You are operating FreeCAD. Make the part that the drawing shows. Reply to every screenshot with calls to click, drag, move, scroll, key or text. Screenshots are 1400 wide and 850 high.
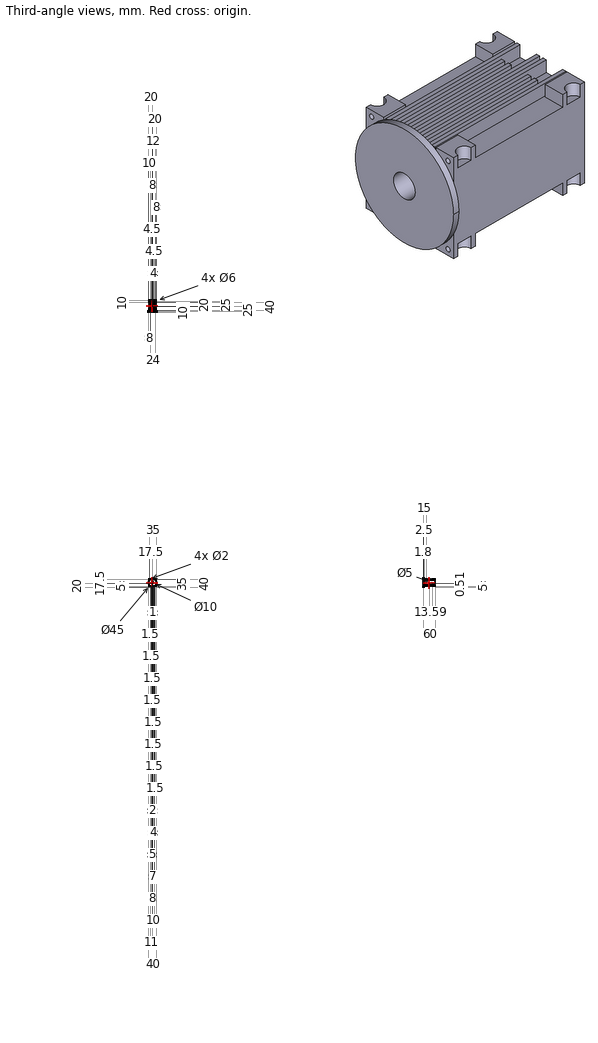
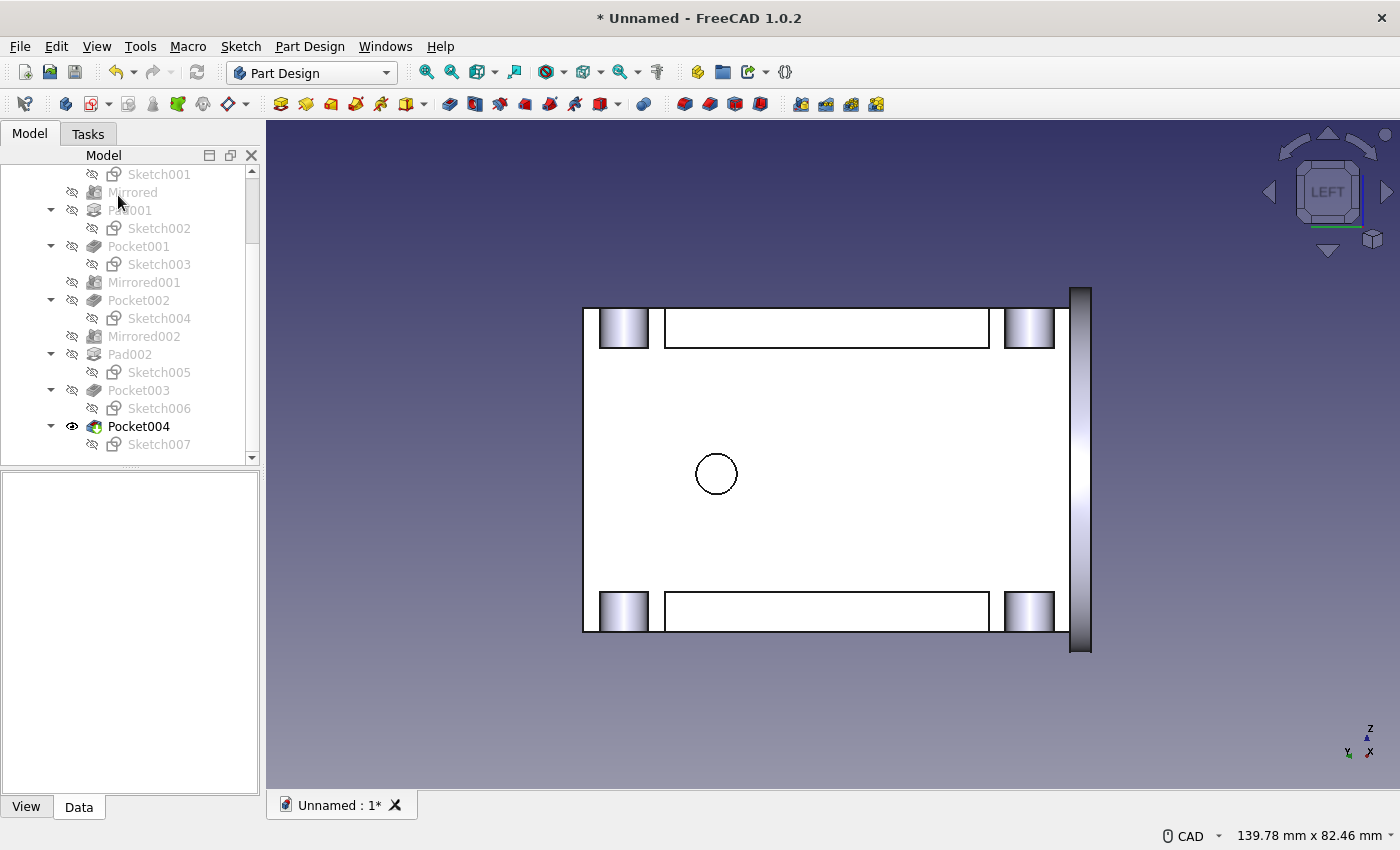
key(4)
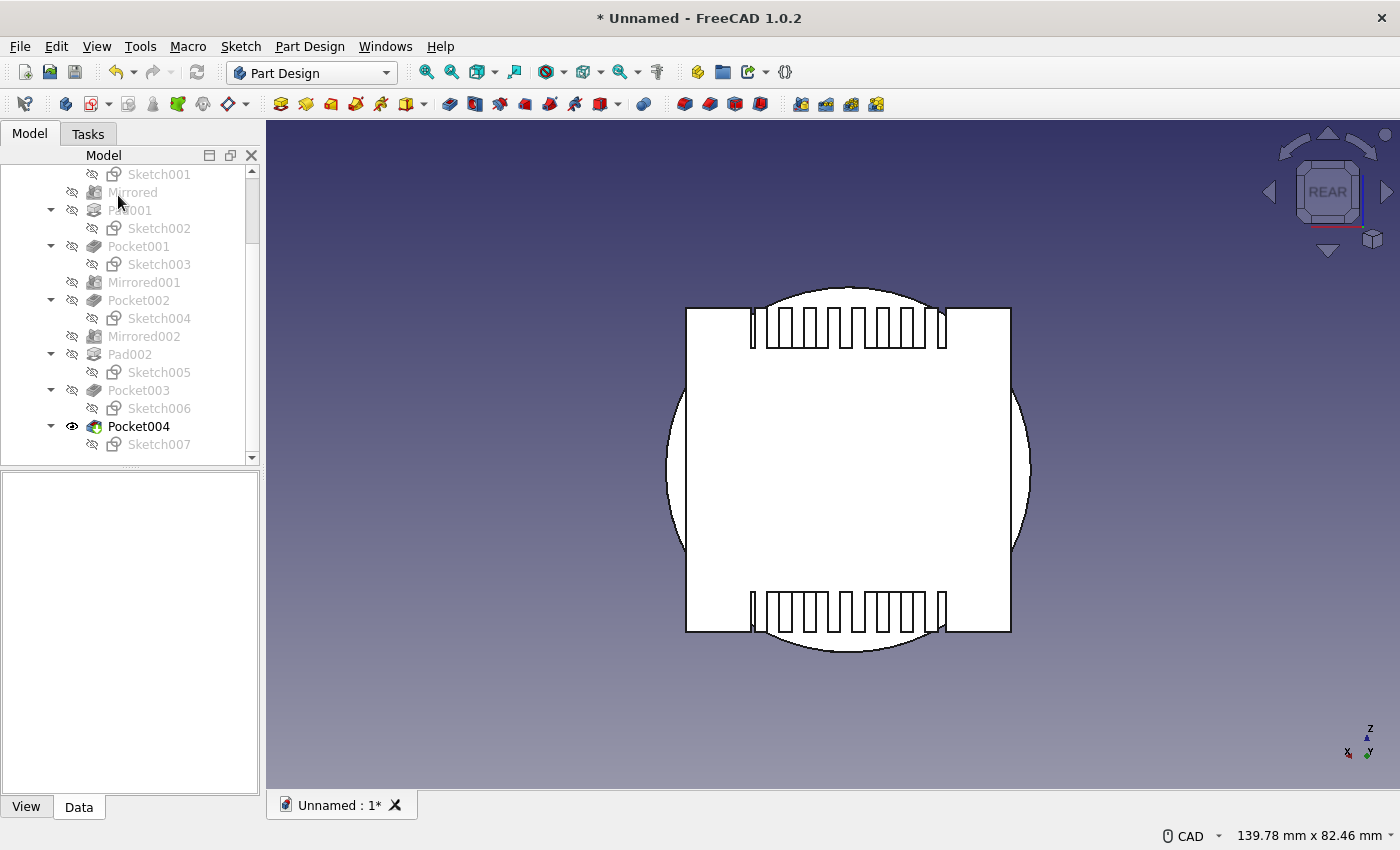
click(896, 299)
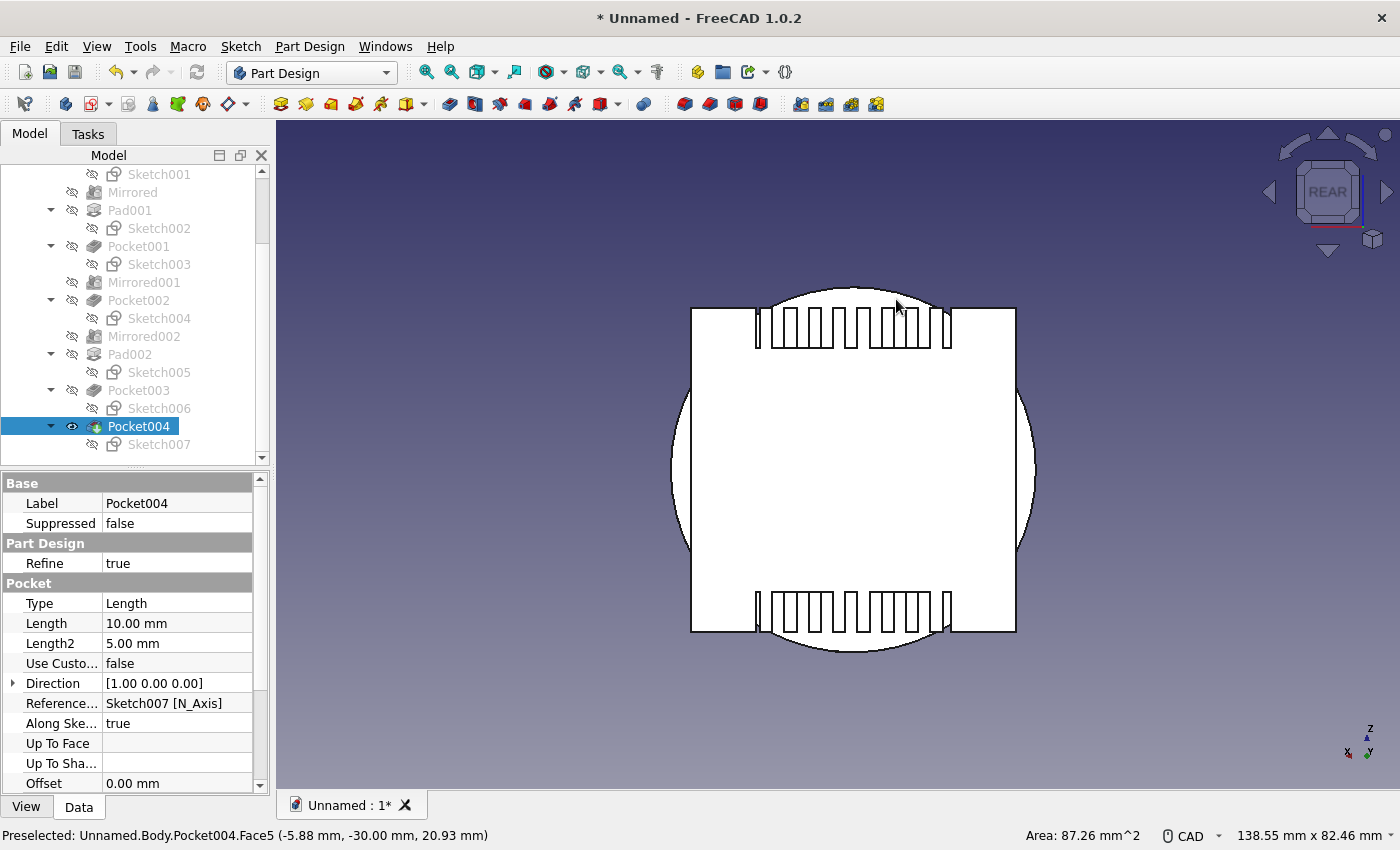
click(90, 104)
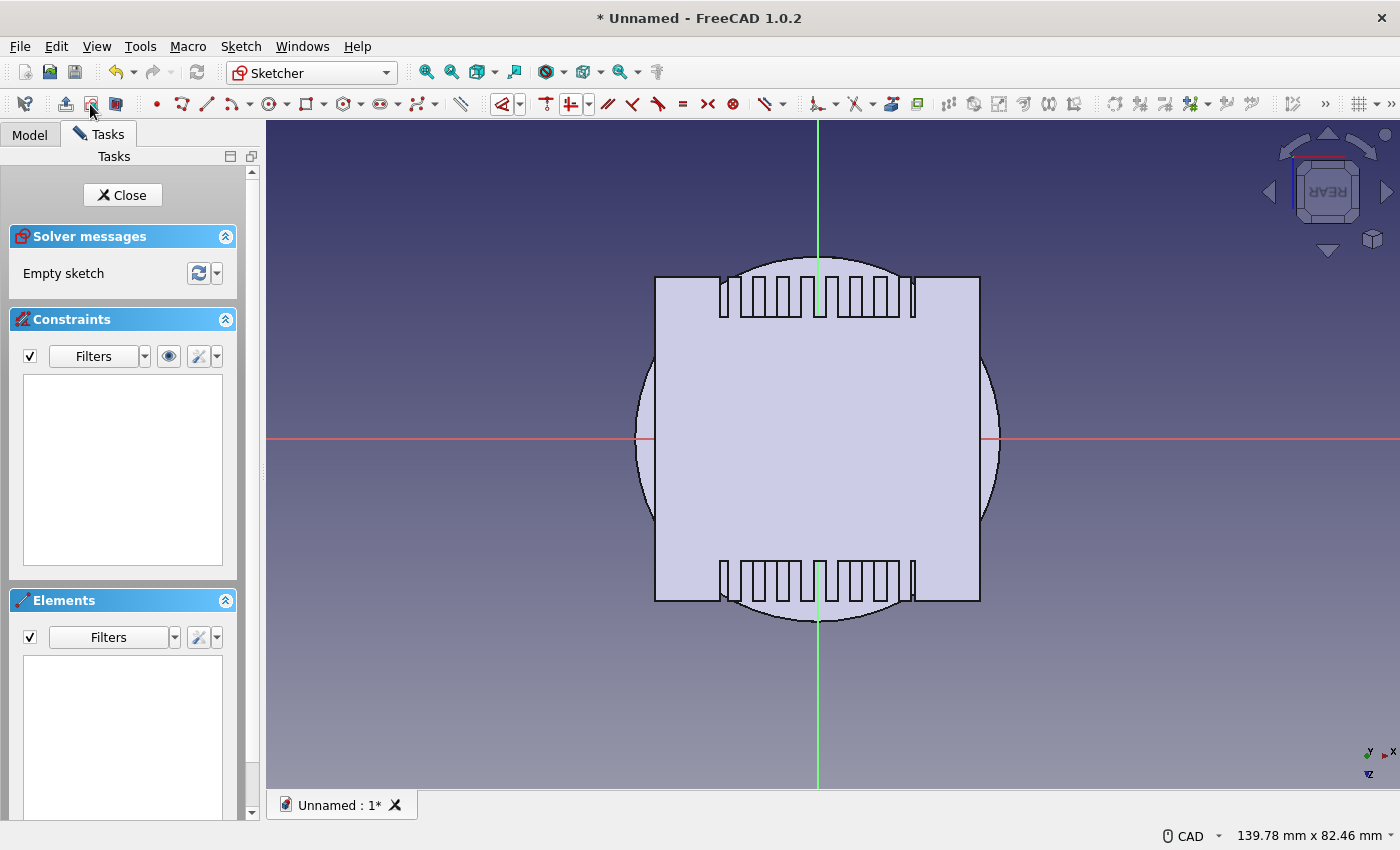
scroll(926, 408, up, 2)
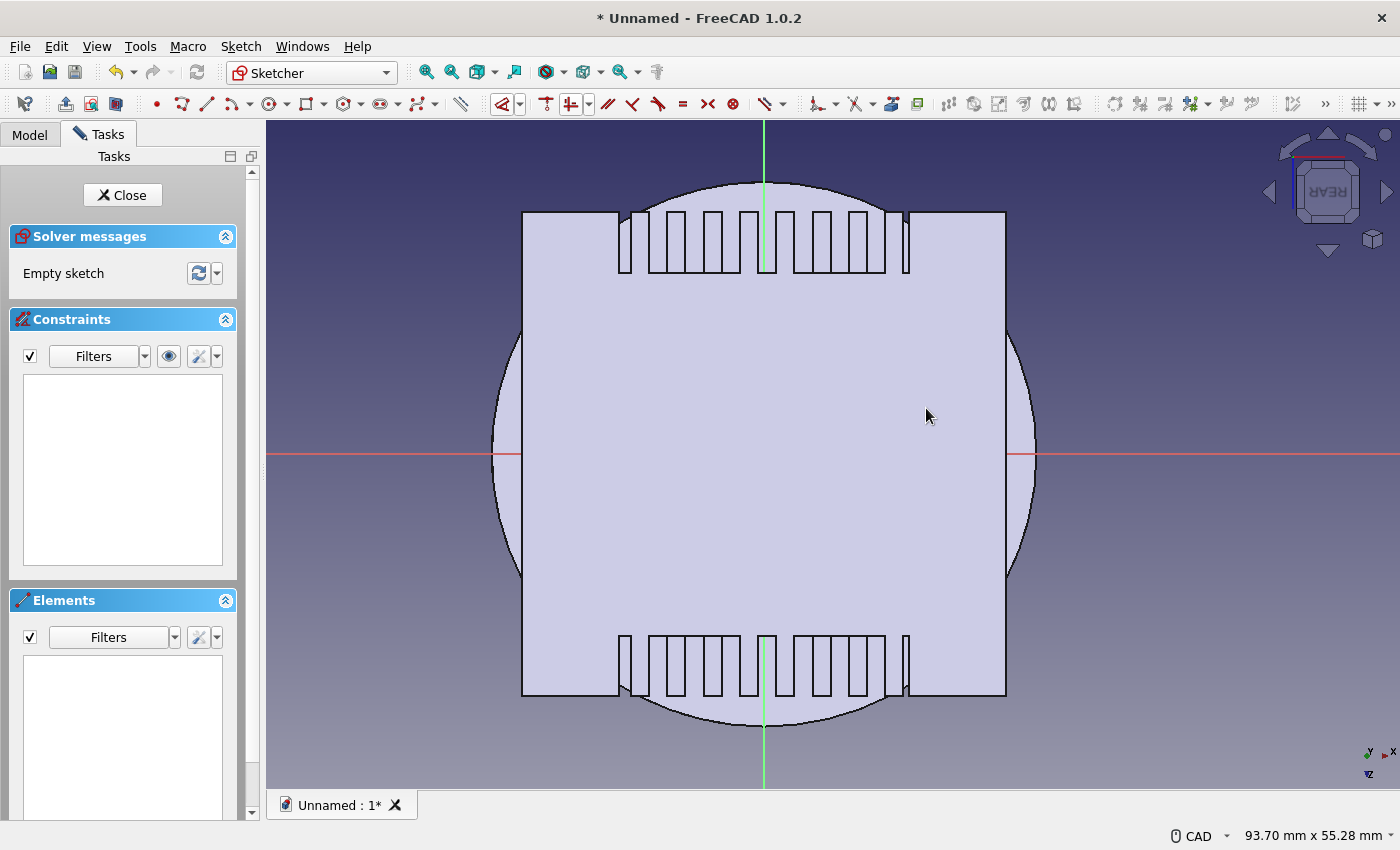
click(268, 104)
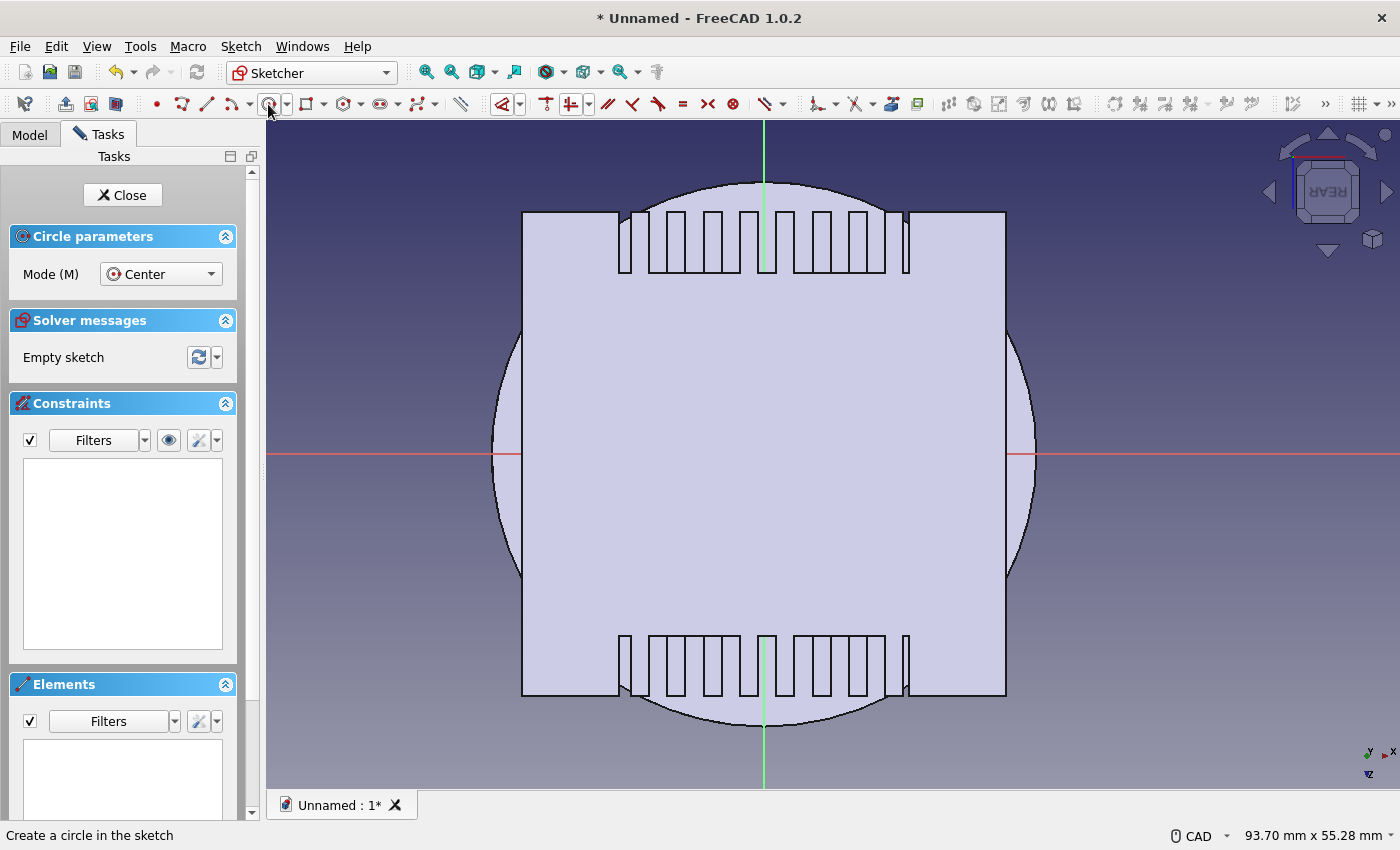
scroll(552, 666, up, 4)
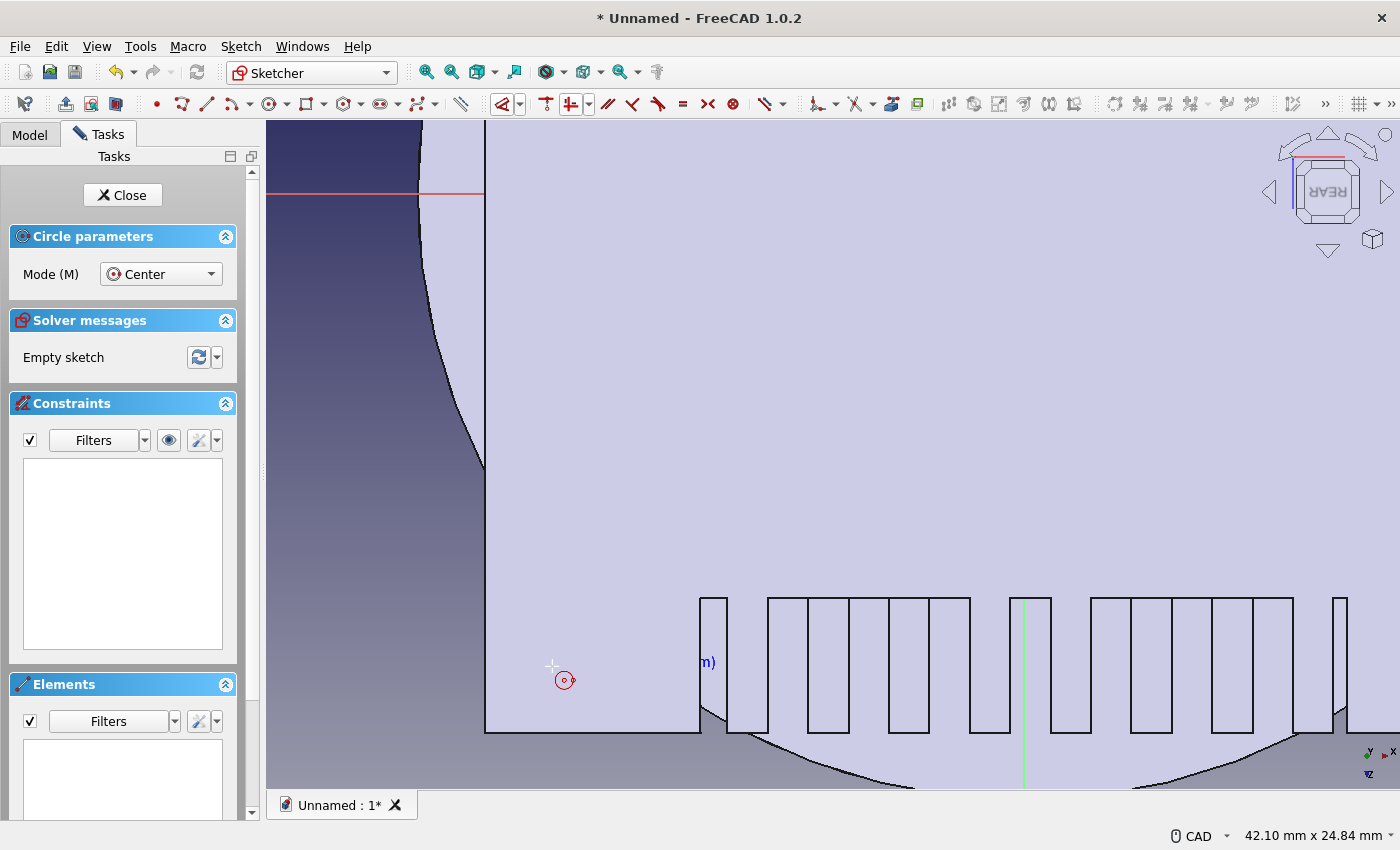
click(552, 665)
click(571, 646)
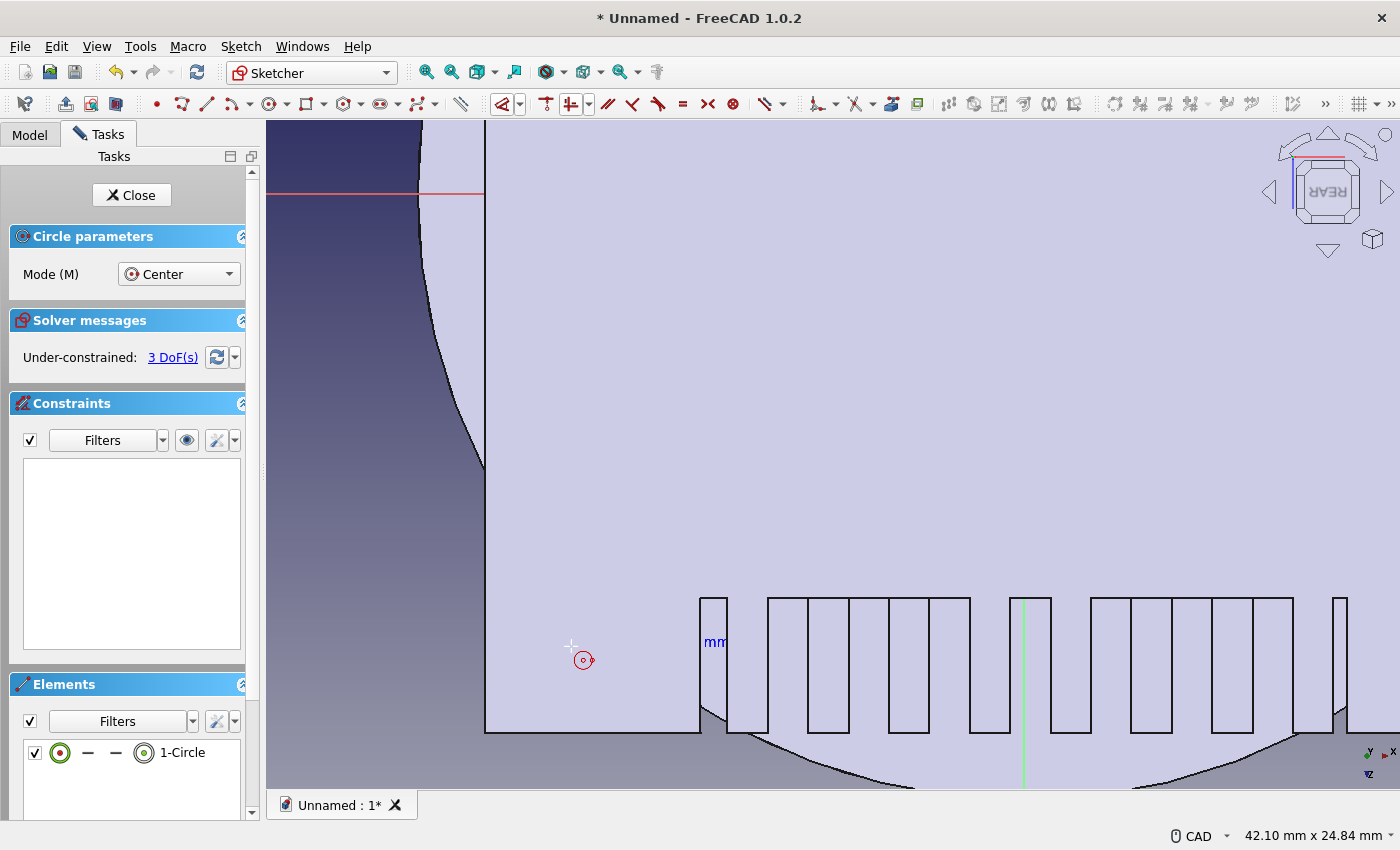
scroll(553, 667, down, 4)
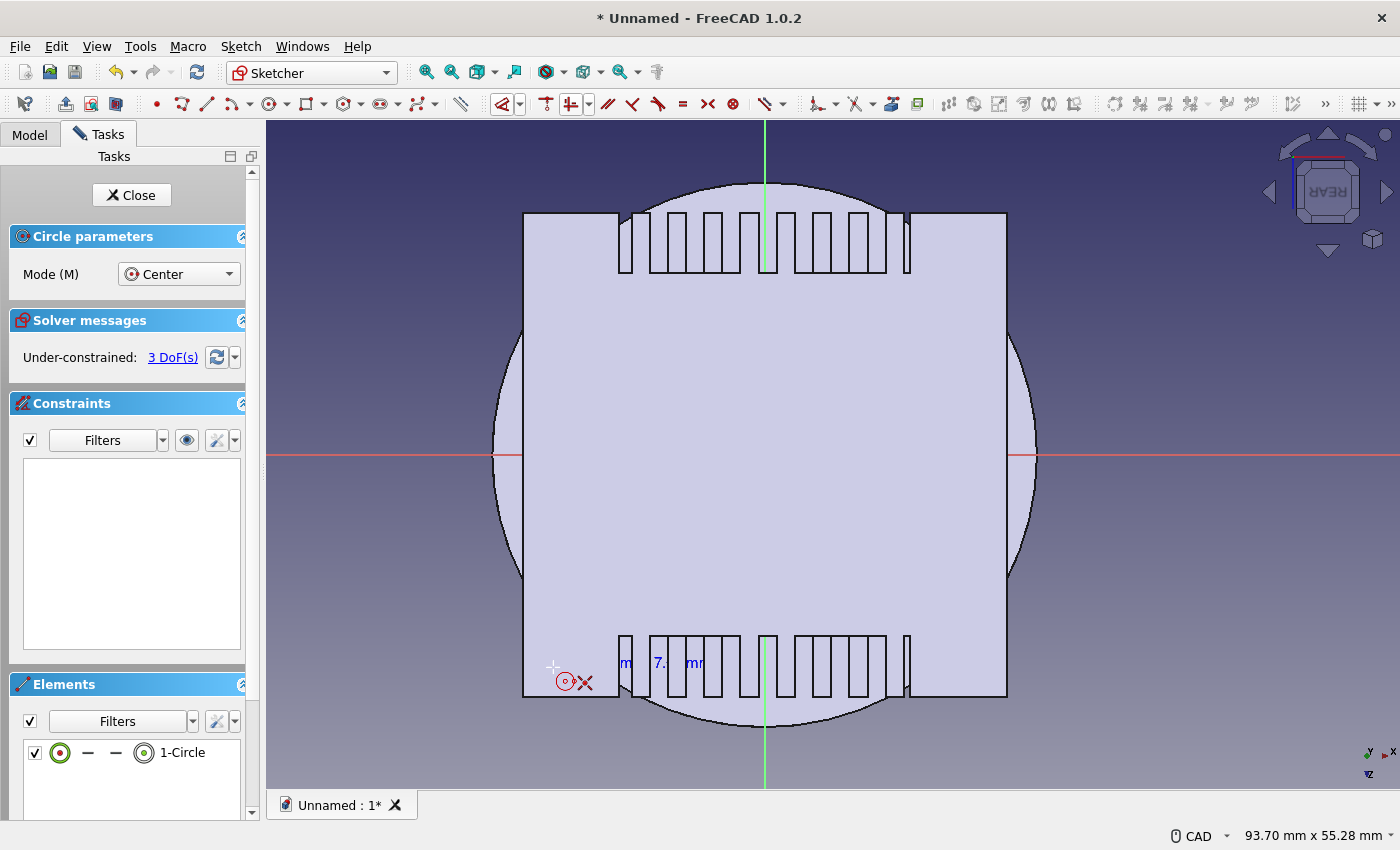
scroll(976, 667, up, 4)